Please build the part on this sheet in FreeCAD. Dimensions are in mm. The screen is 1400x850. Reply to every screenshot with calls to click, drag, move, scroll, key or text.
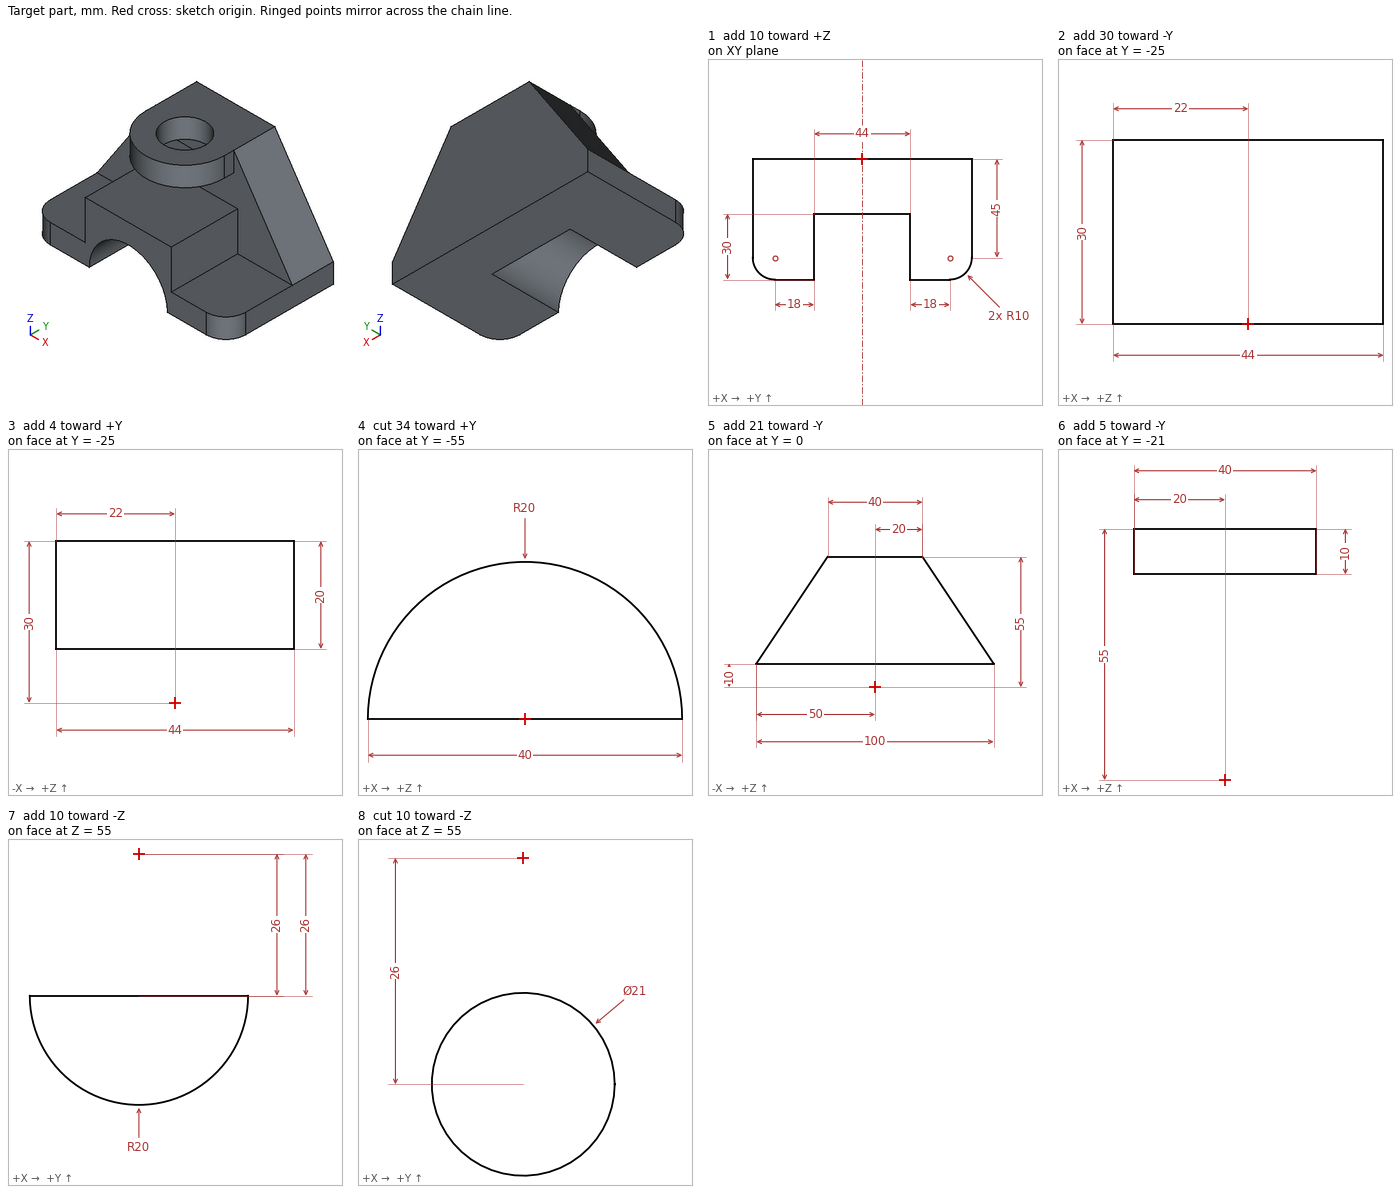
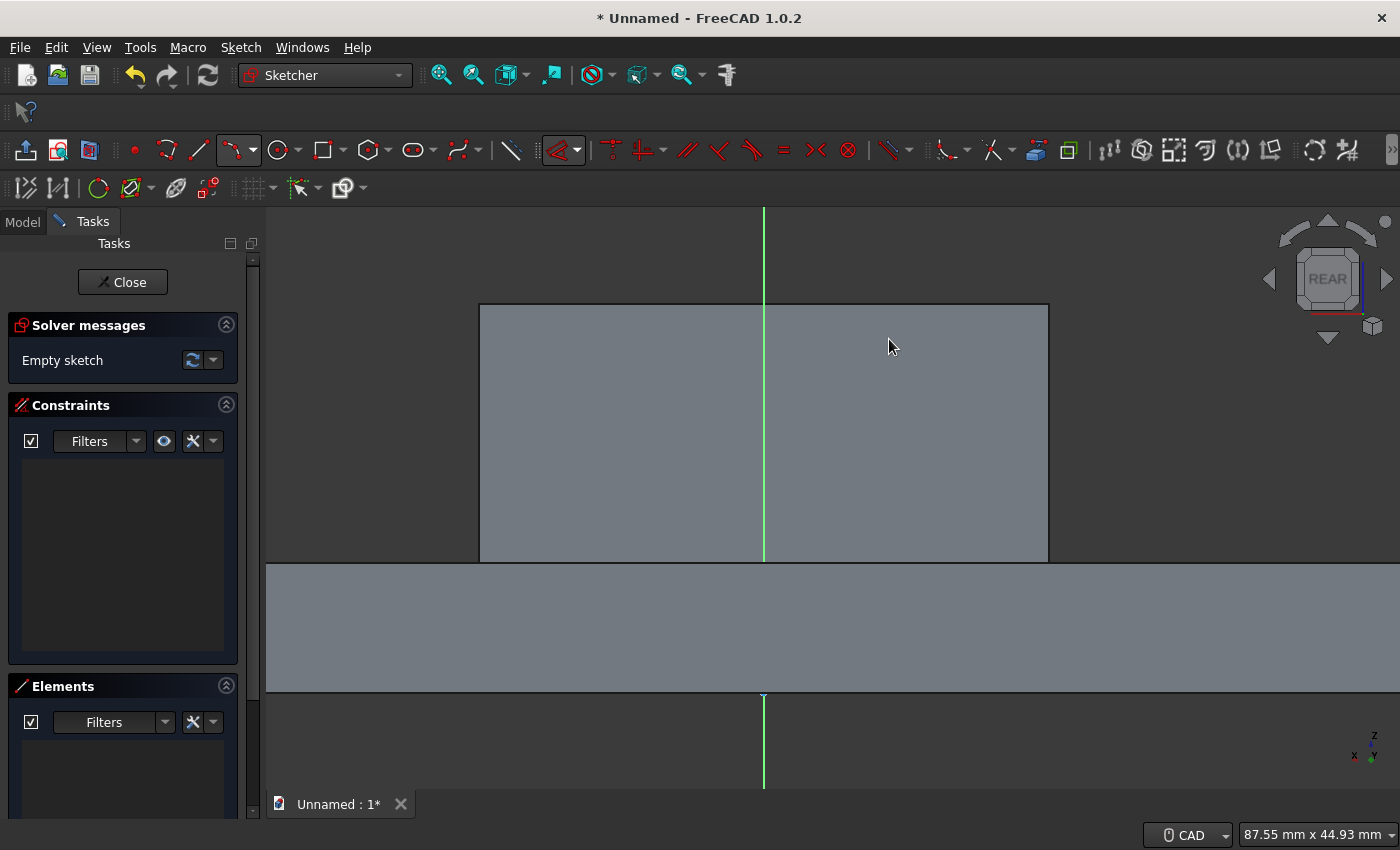
click(324, 150)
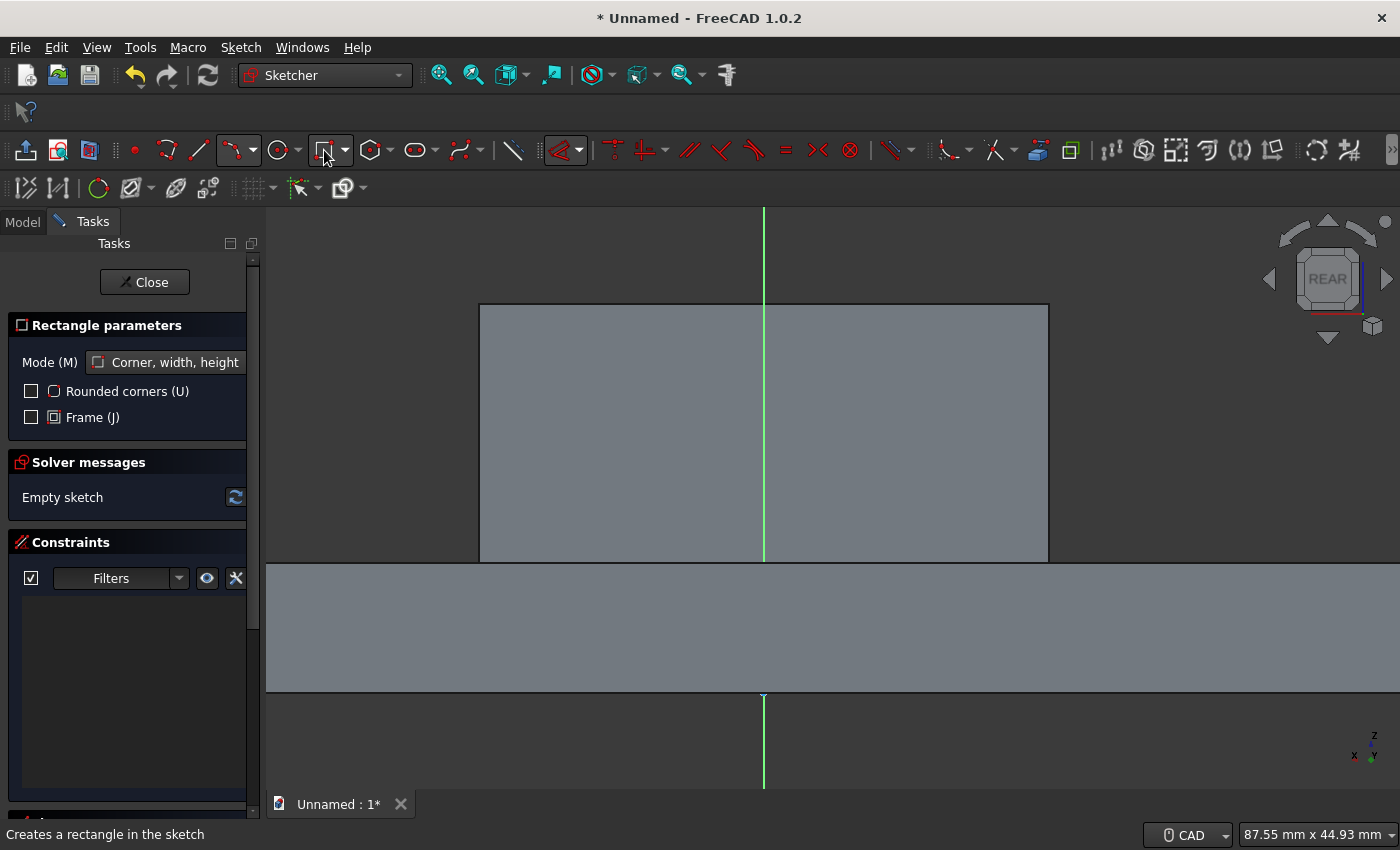
click(479, 304)
move(1049, 563)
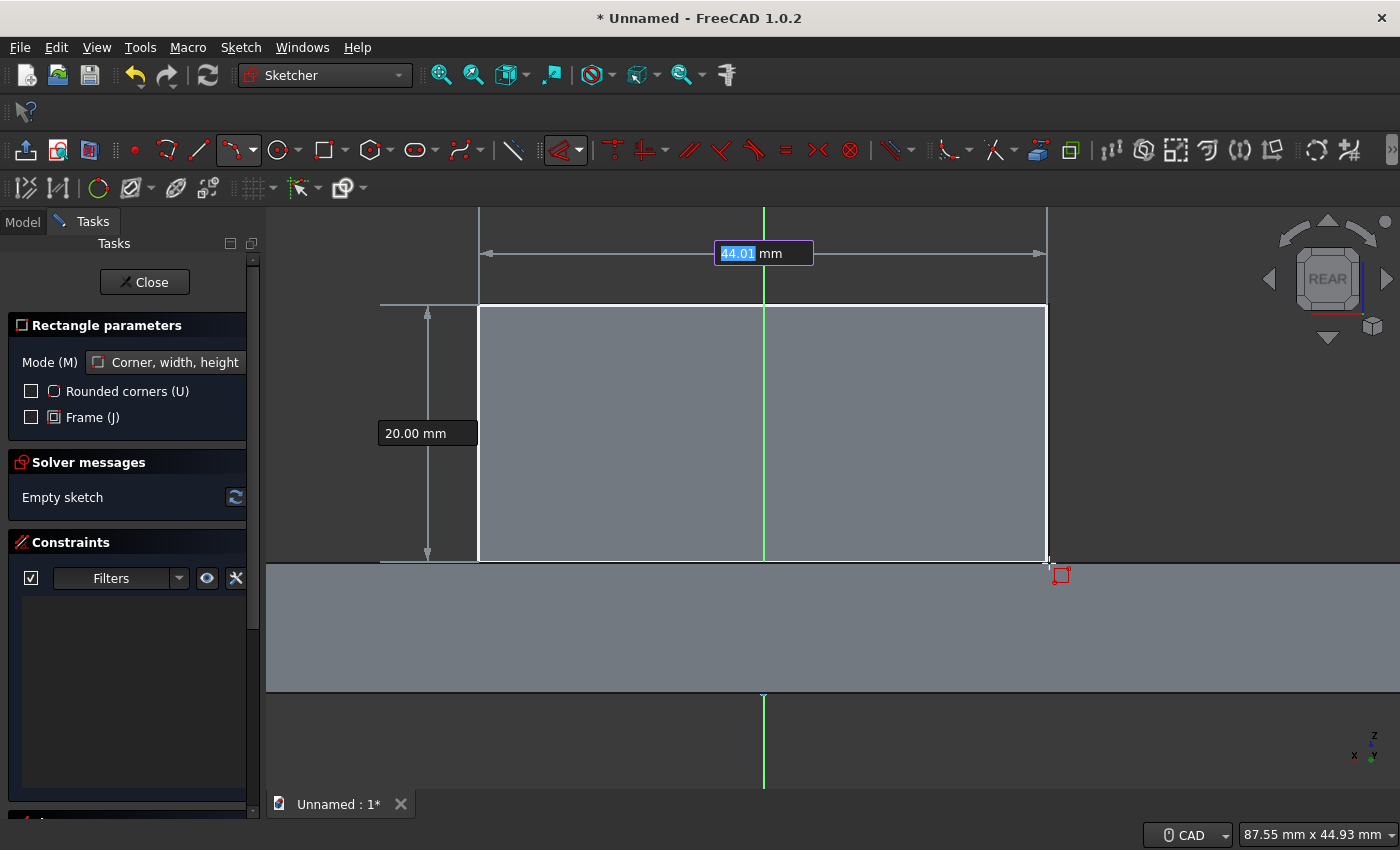
text(44)
key(Tab)
text(20)
key(Return)
key(Escape)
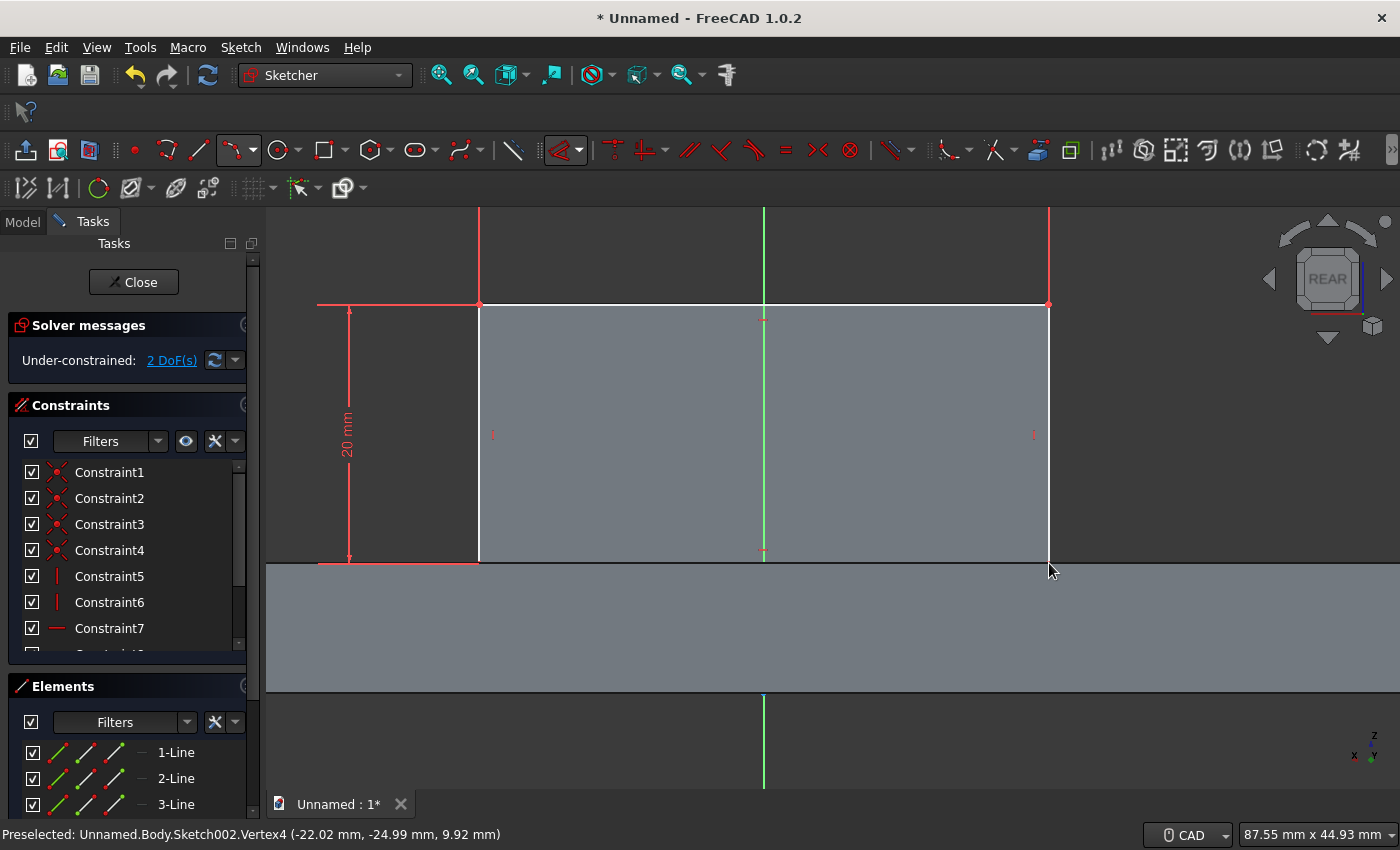
click(479, 305)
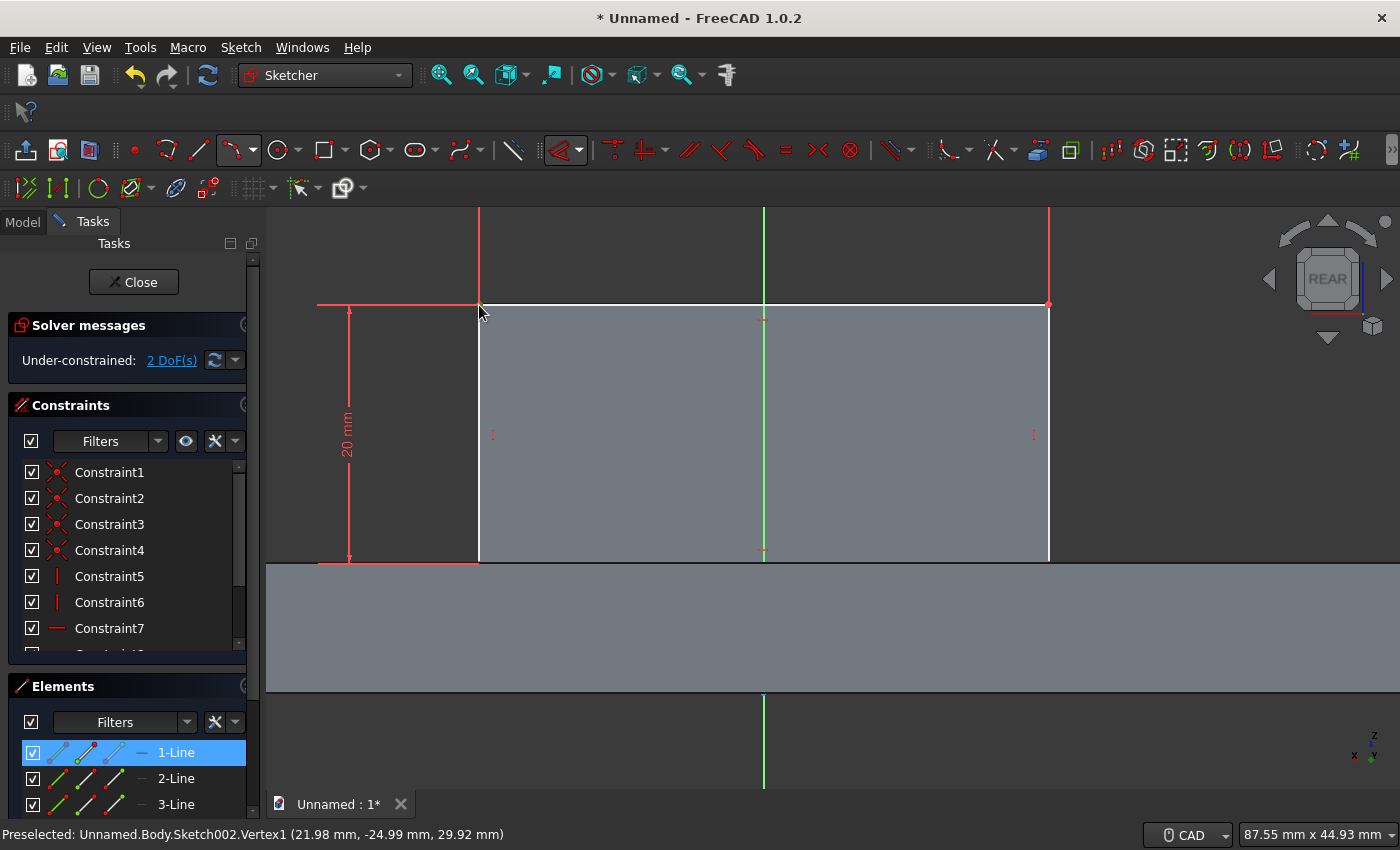
click(582, 150)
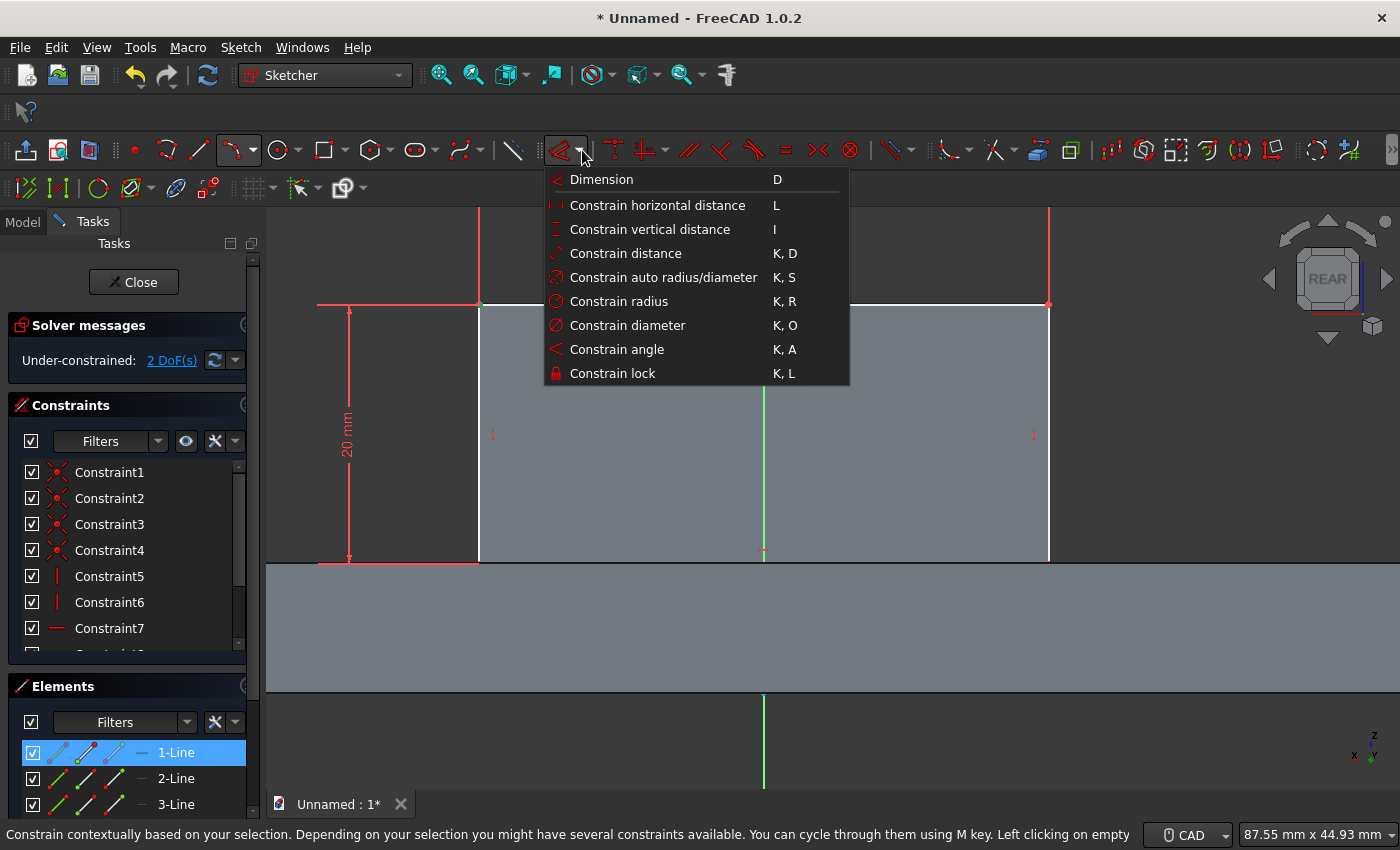
click(697, 205)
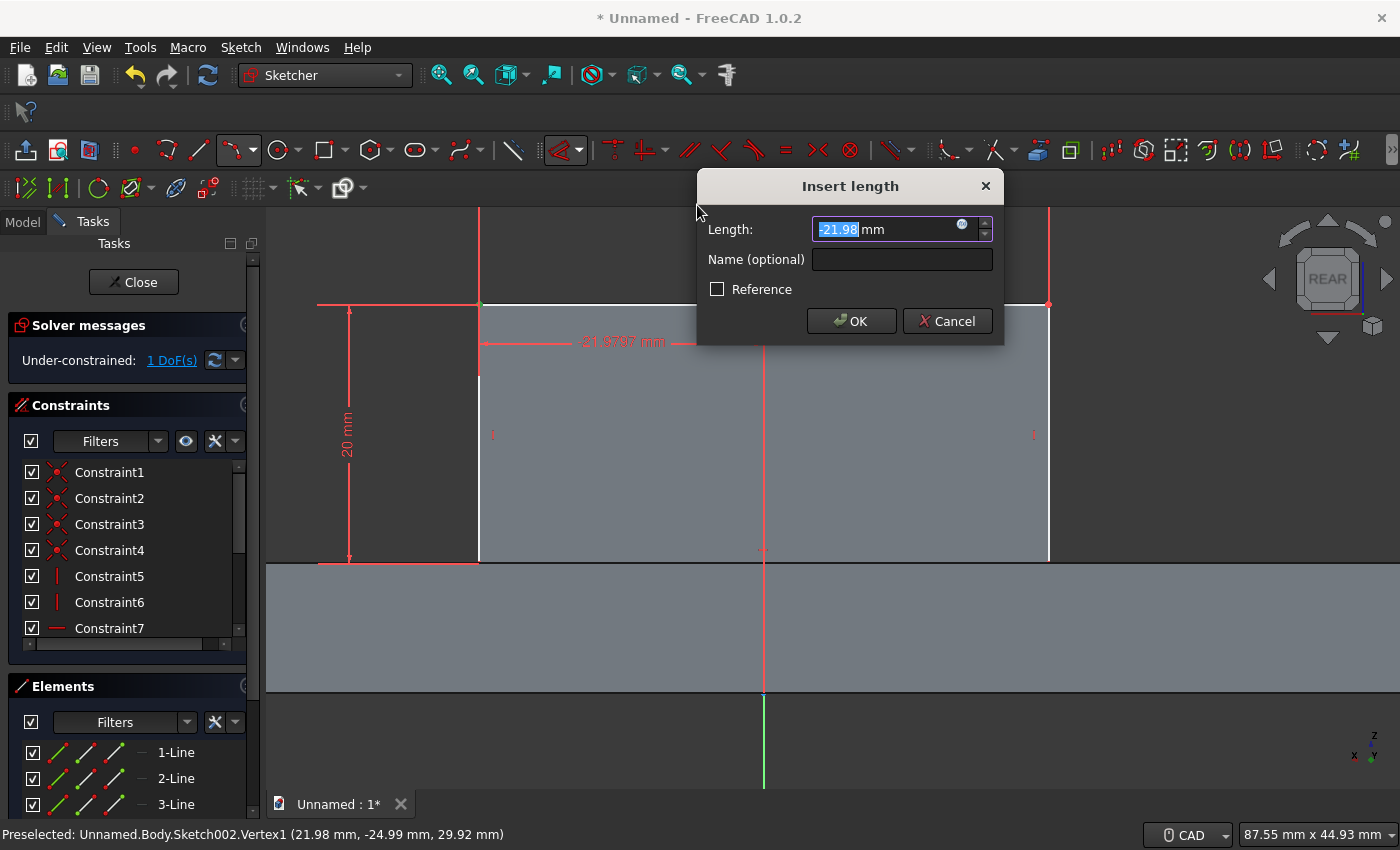
text(-22)
key(Return)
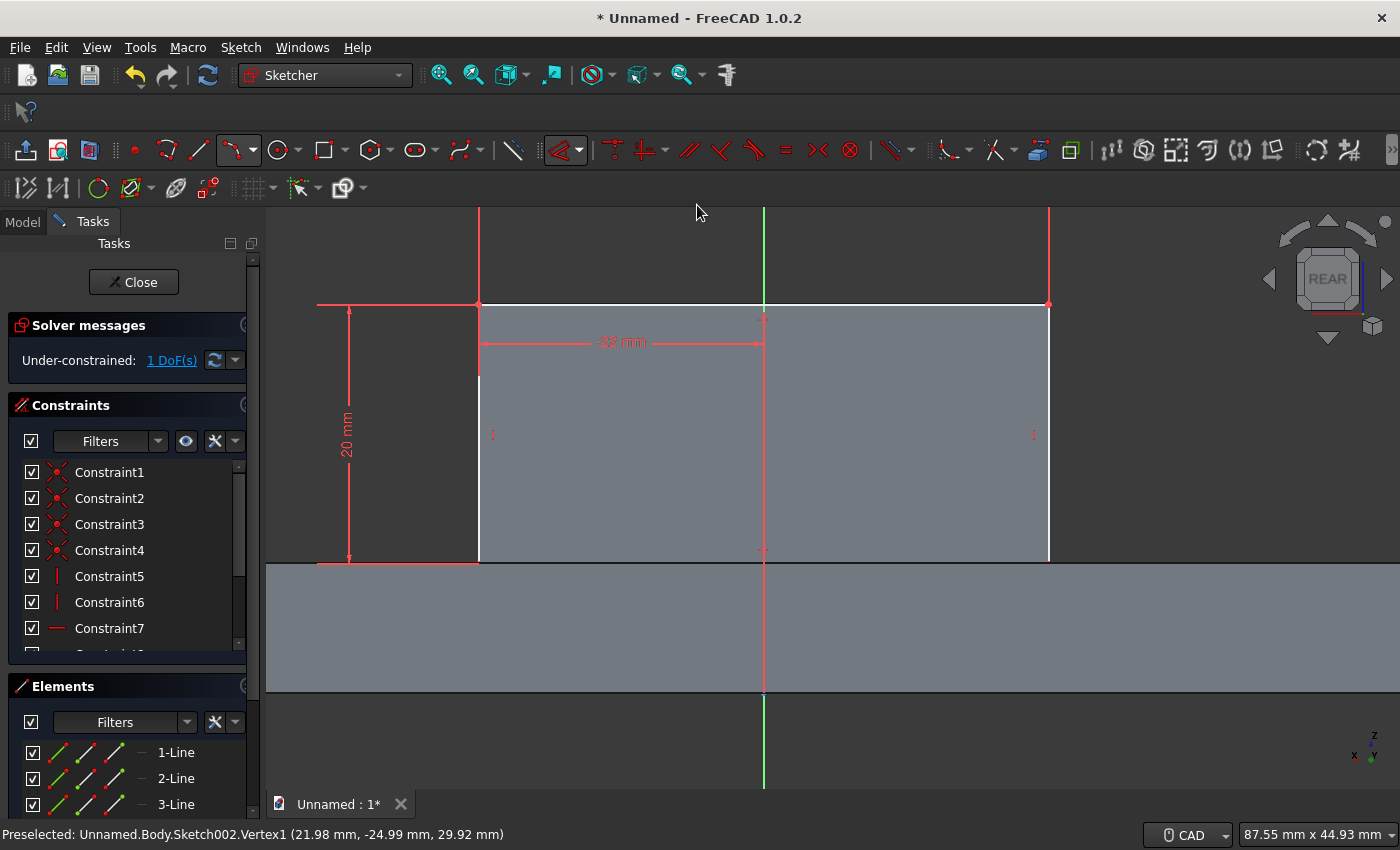
click(479, 305)